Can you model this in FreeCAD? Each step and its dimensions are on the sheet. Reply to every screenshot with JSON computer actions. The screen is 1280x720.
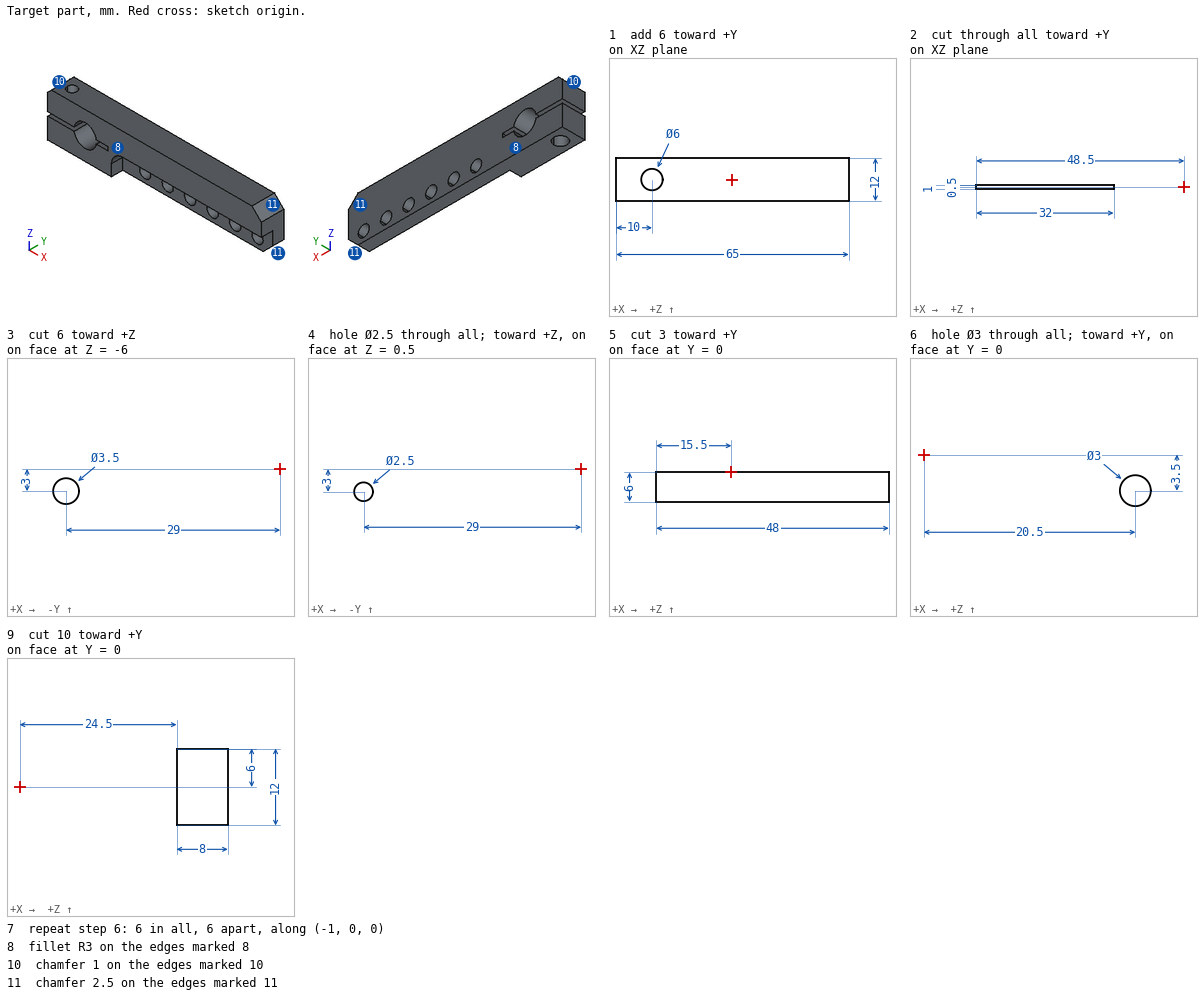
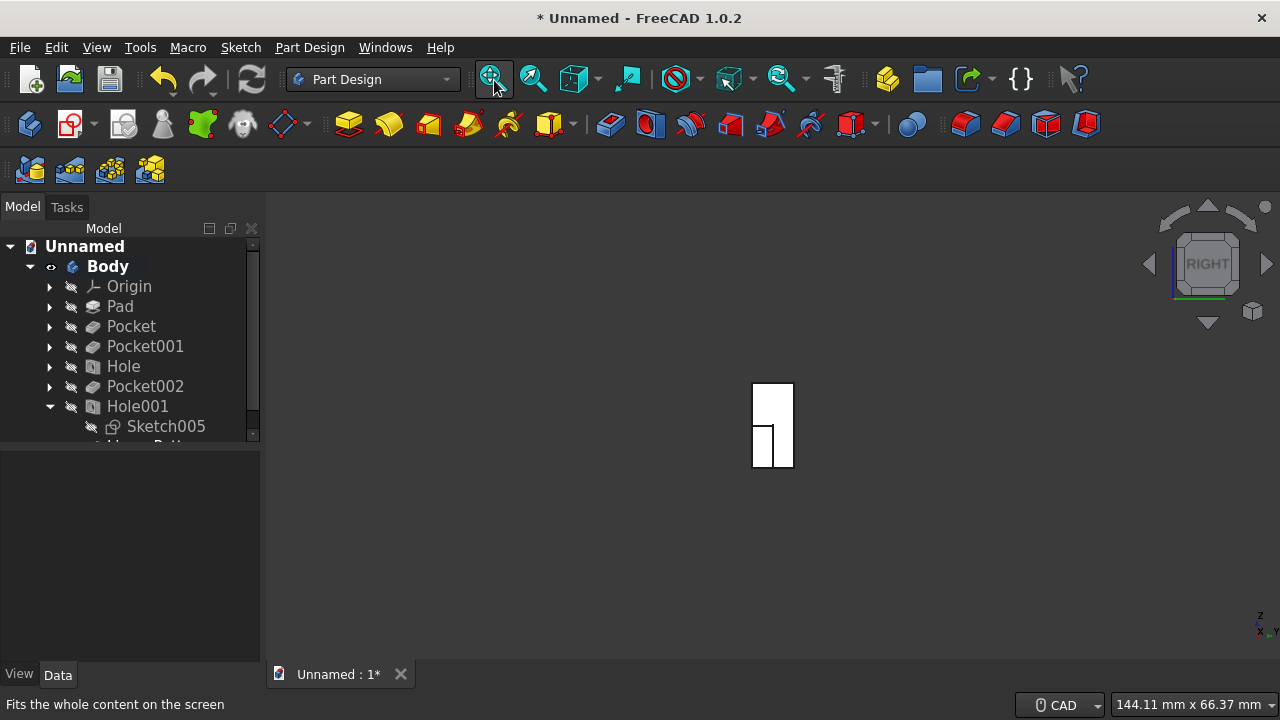
{"action": "key", "text": "v f"}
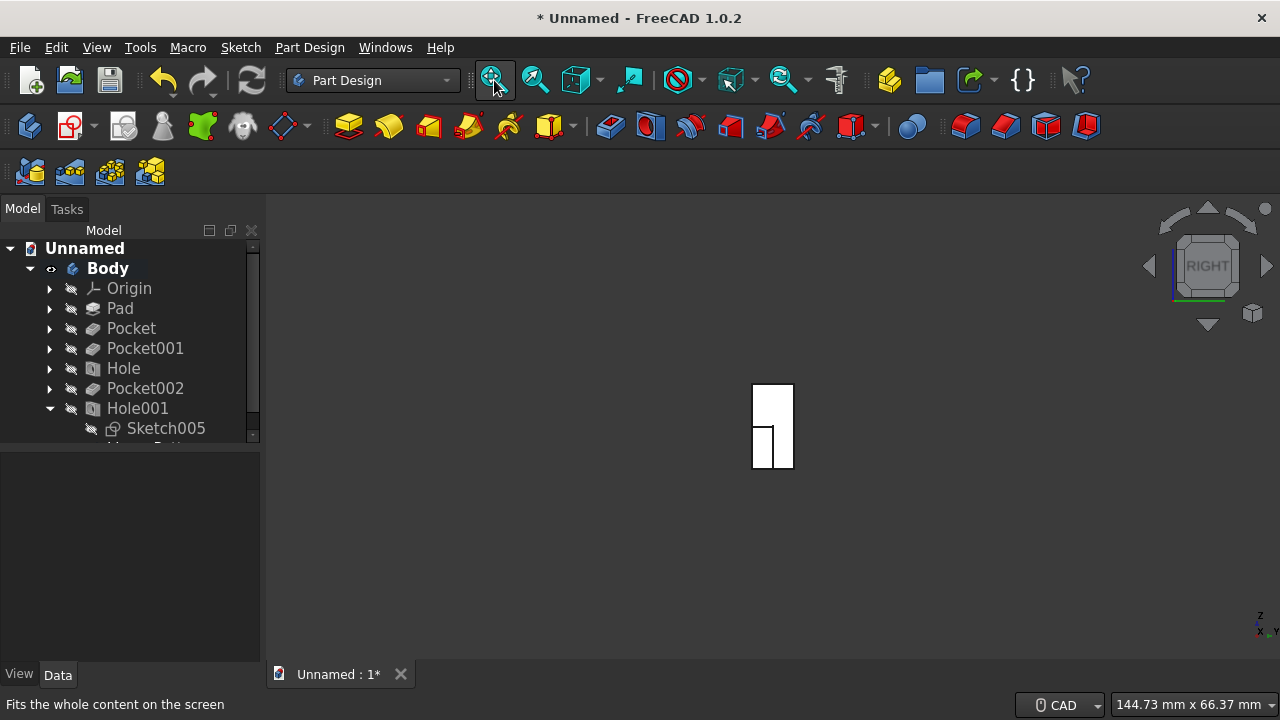
{"action": "scroll", "coordinate": [762, 425], "scroll_direction": "up", "scroll_amount": 4}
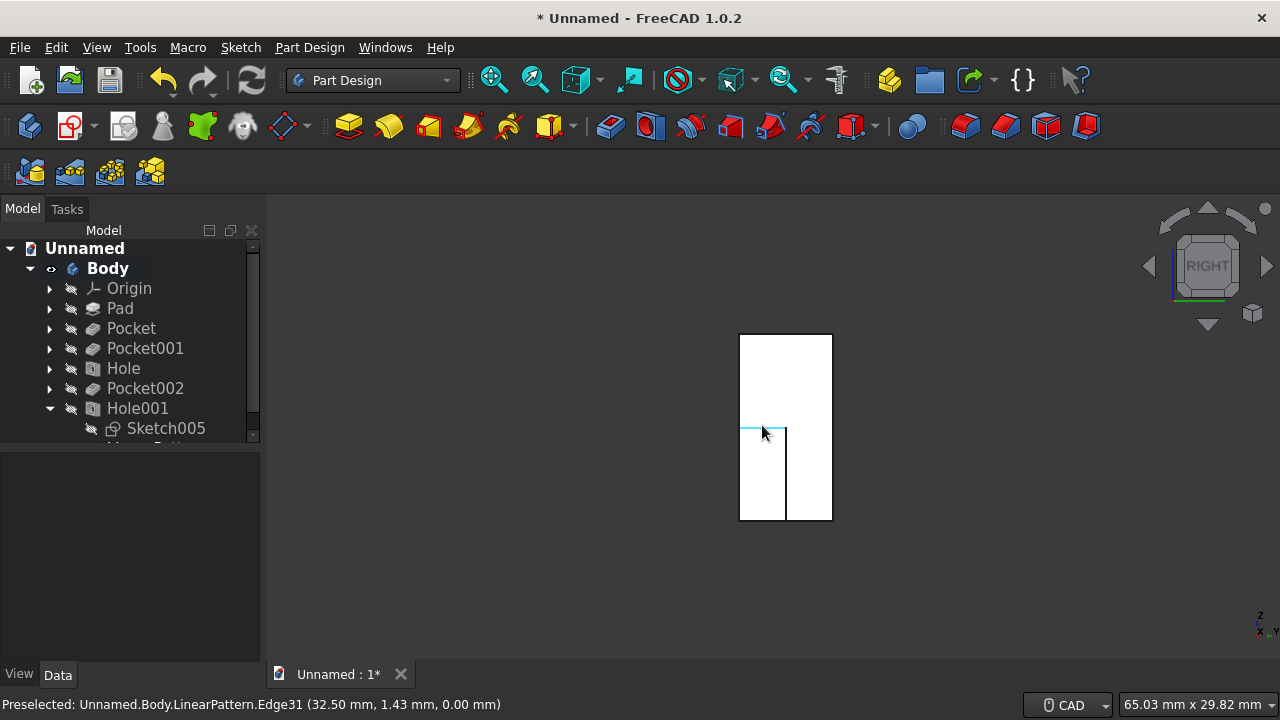
{"action": "left_click", "coordinate": [496, 80]}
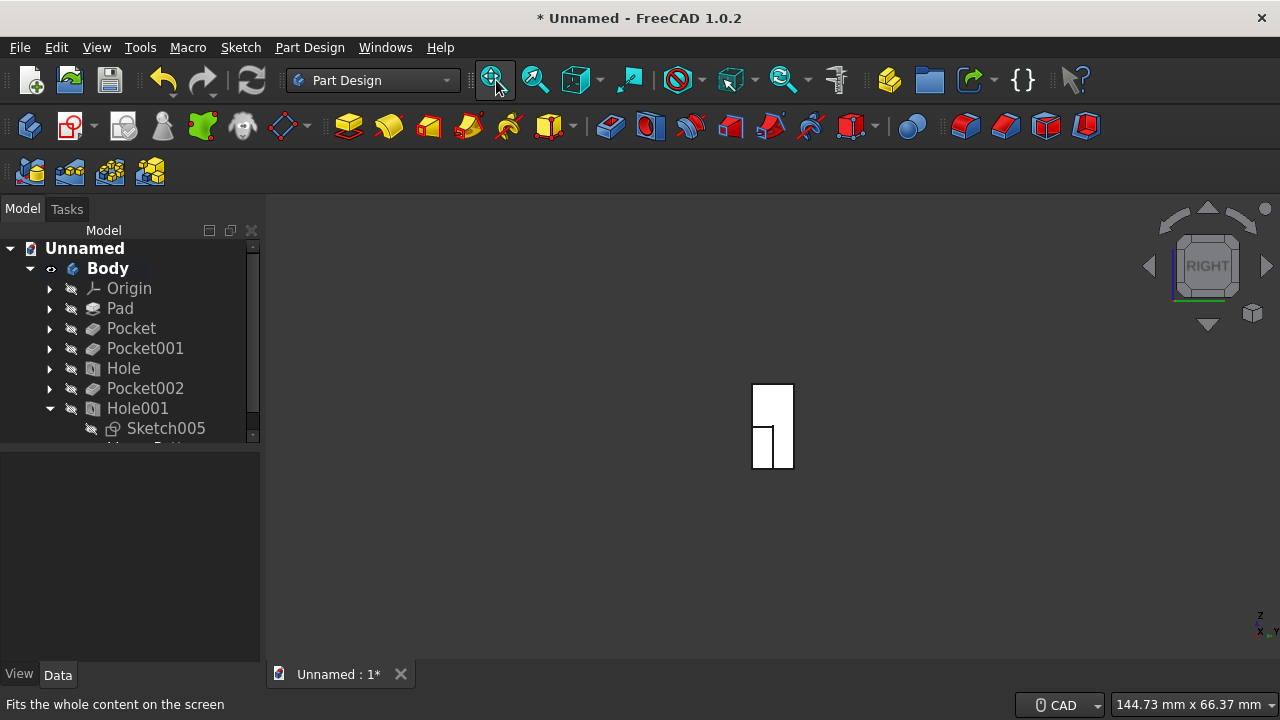
{"action": "key", "text": "5"}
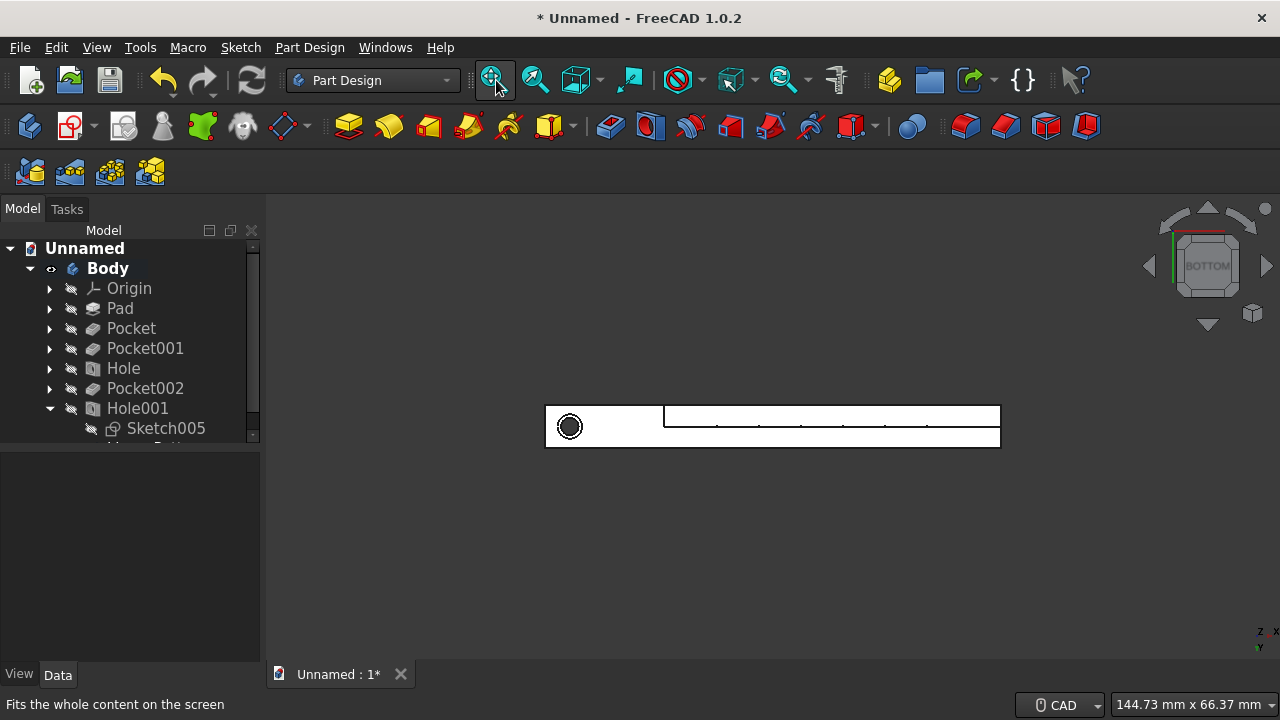
{"action": "left_click", "coordinate": [496, 80]}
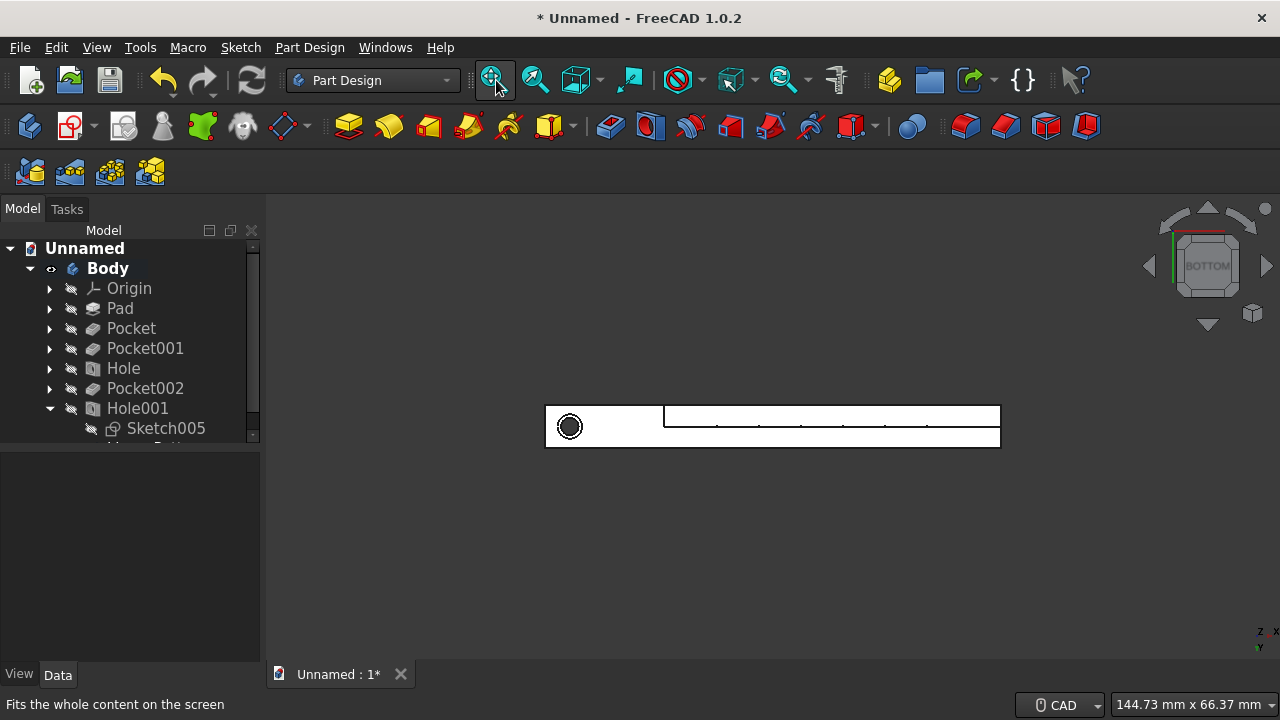
{"action": "scroll", "coordinate": [664, 415], "scroll_direction": "up", "scroll_amount": 4}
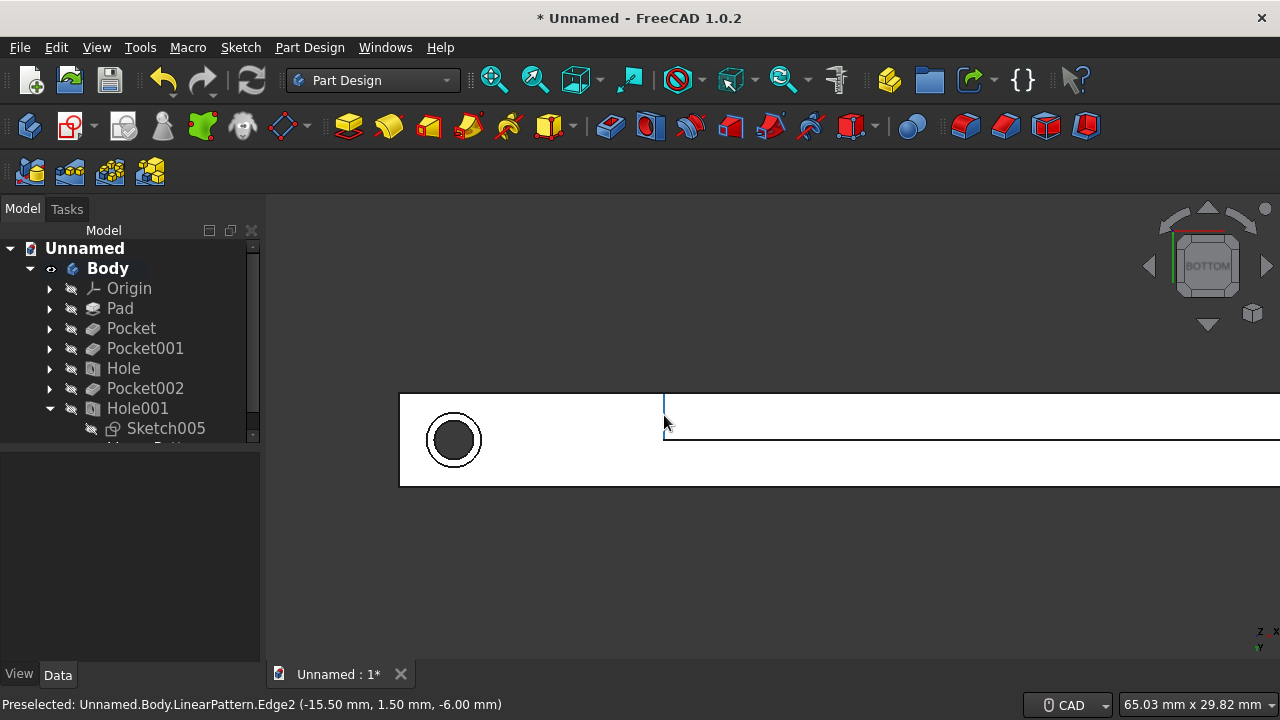
{"action": "left_click", "coordinate": [496, 80]}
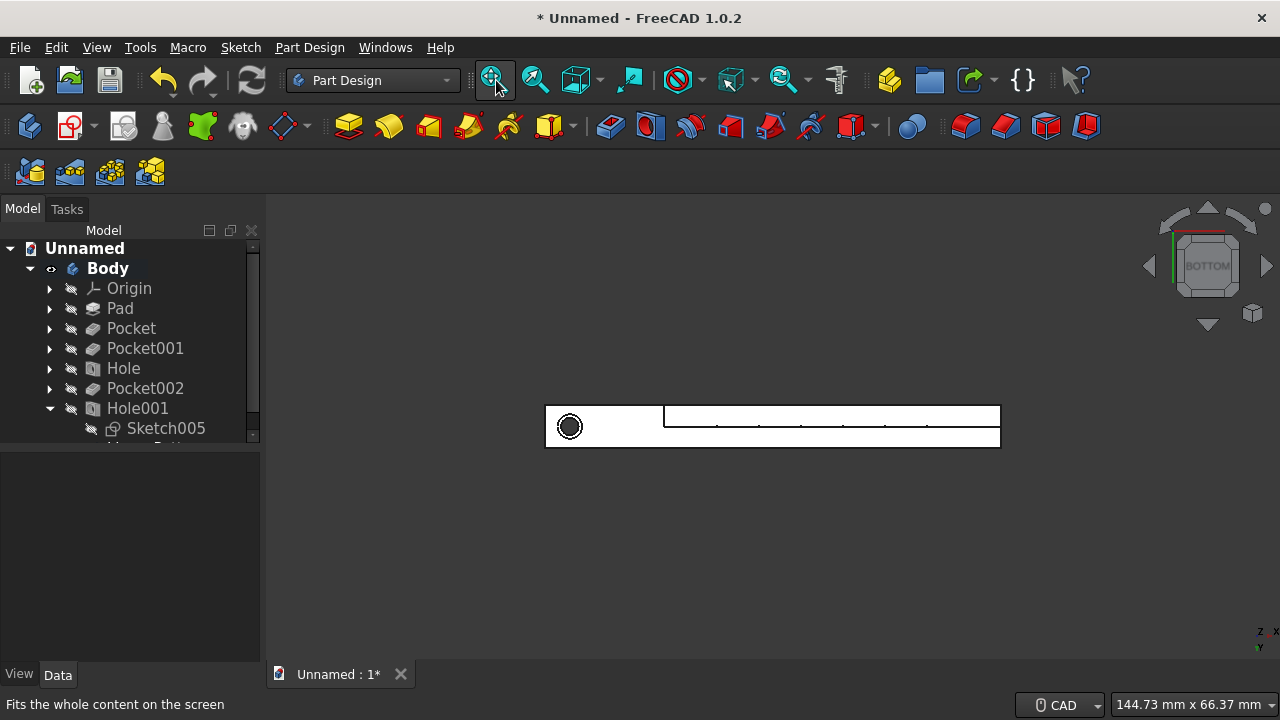
{"action": "key", "text": "4"}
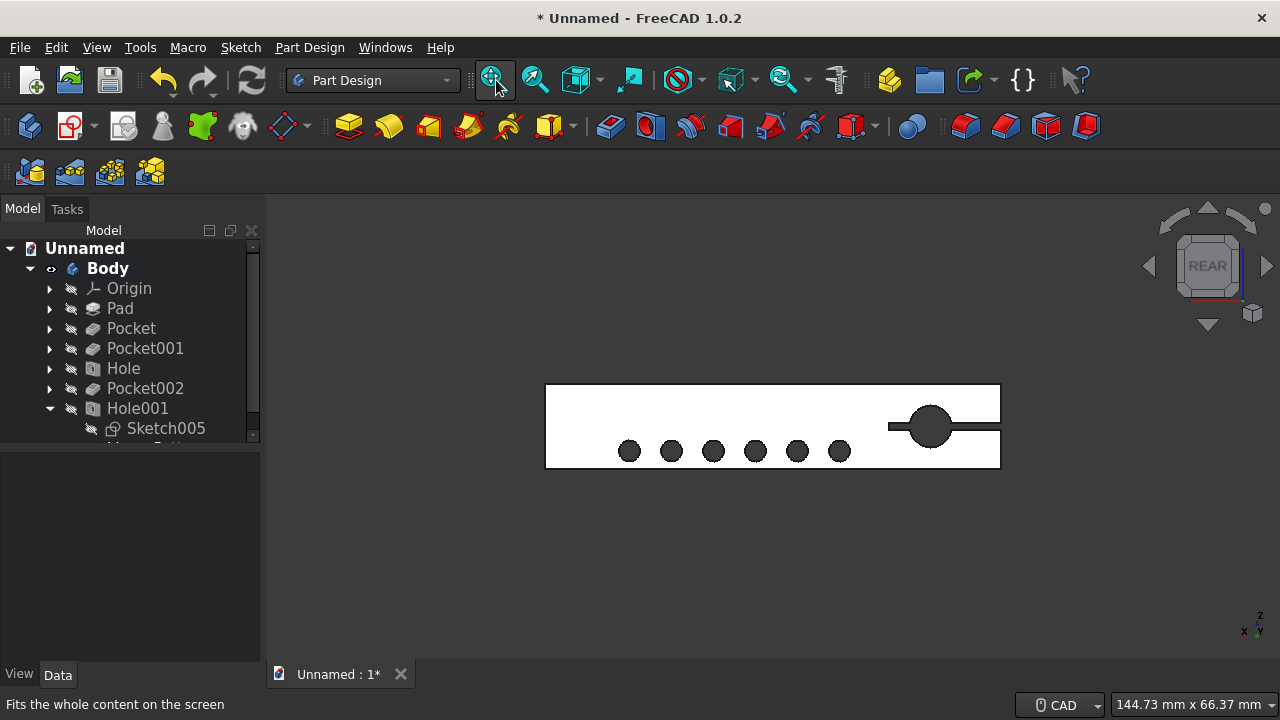
{"action": "left_click", "coordinate": [496, 80]}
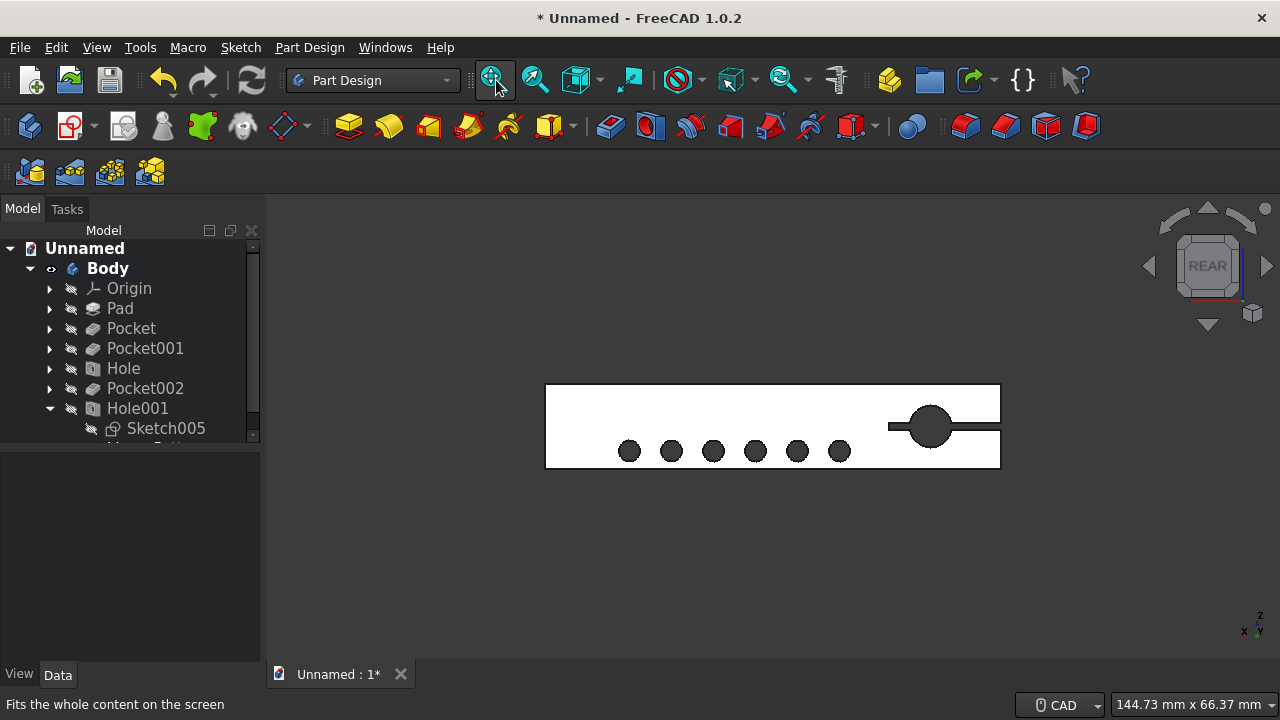
{"action": "scroll", "coordinate": [882, 426], "scroll_direction": "up", "scroll_amount": 4}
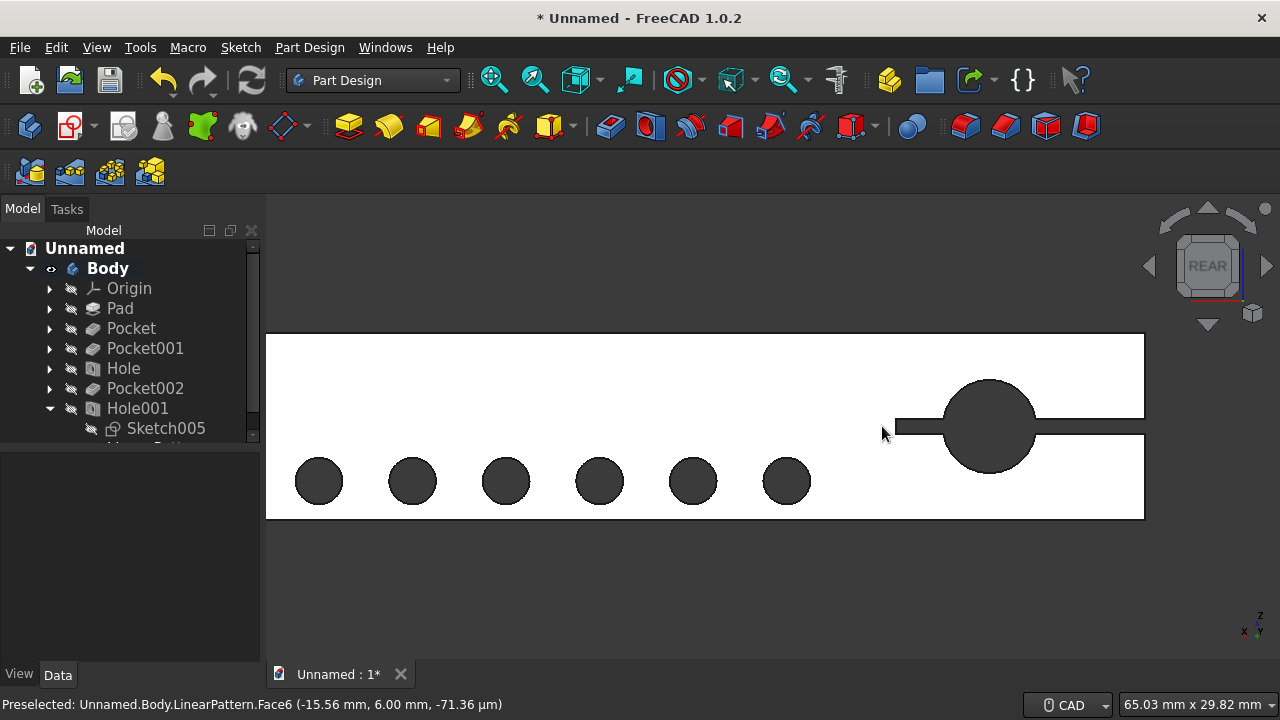
{"action": "left_click", "coordinate": [496, 80]}